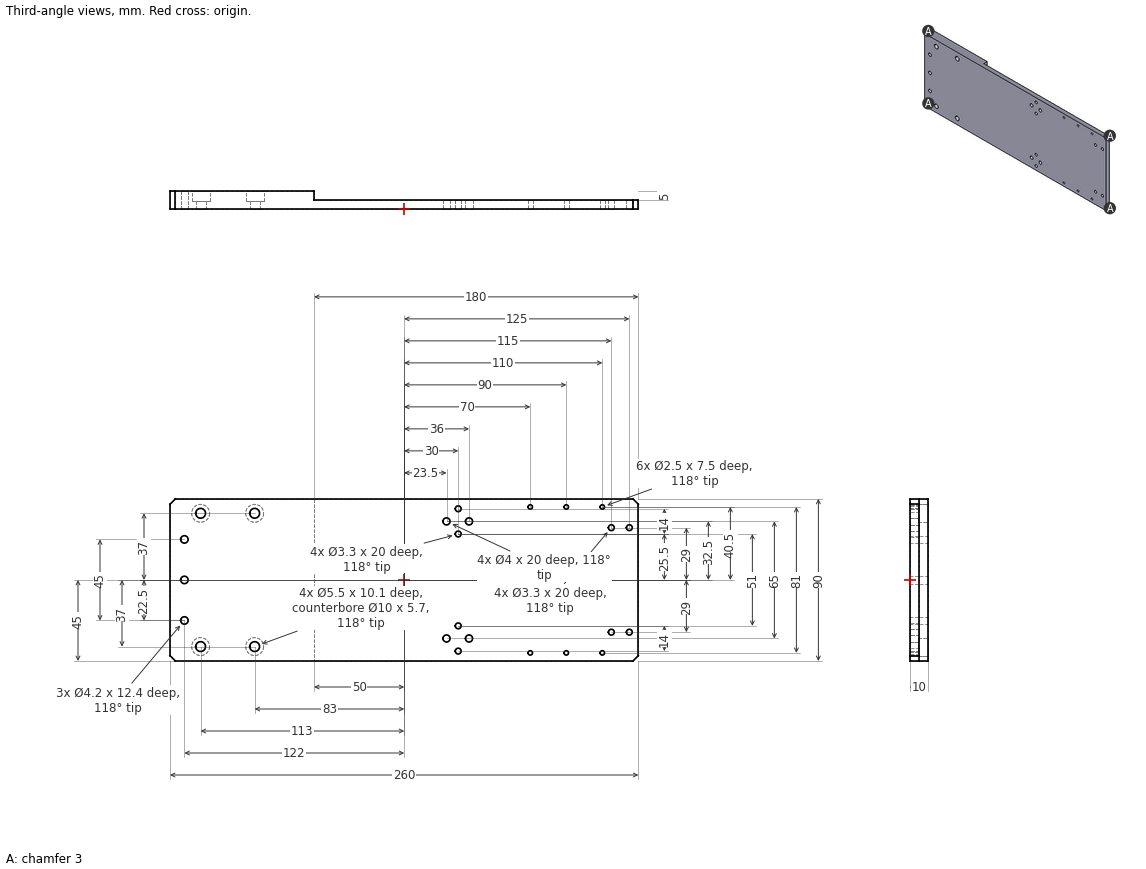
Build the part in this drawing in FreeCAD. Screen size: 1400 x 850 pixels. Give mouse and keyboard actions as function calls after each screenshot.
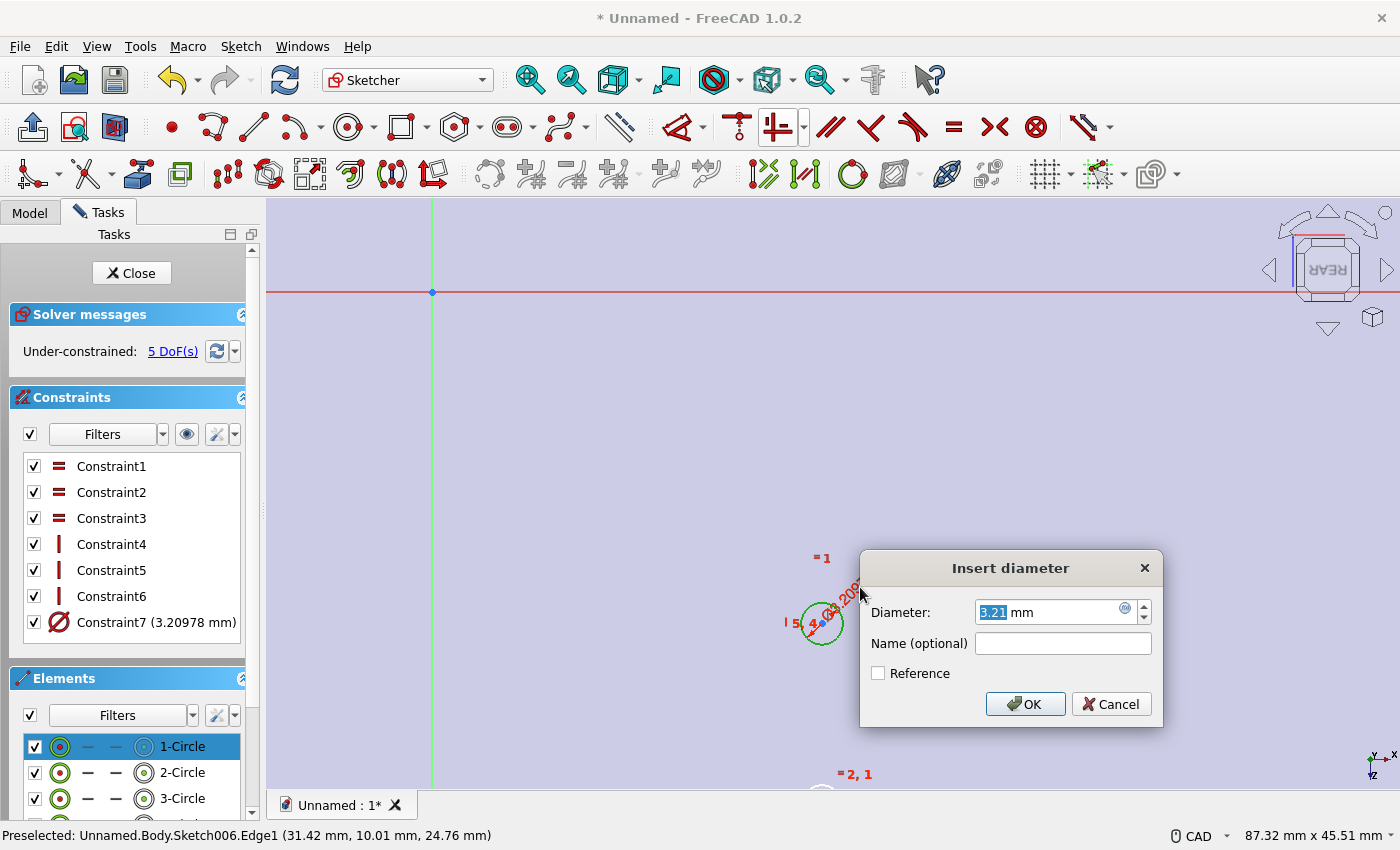
text(3.3)
key(Return)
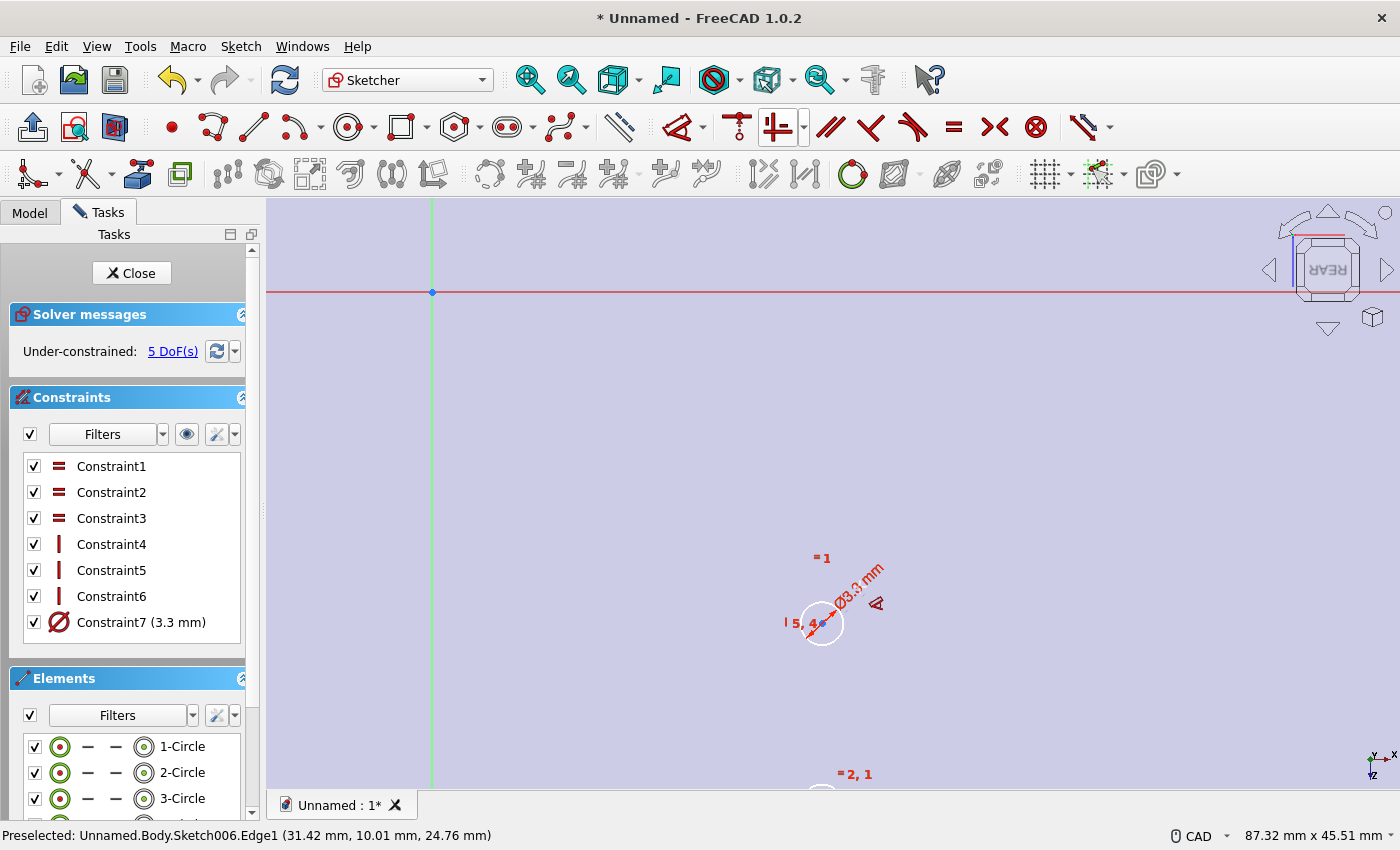
click(822, 624)
click(627, 658)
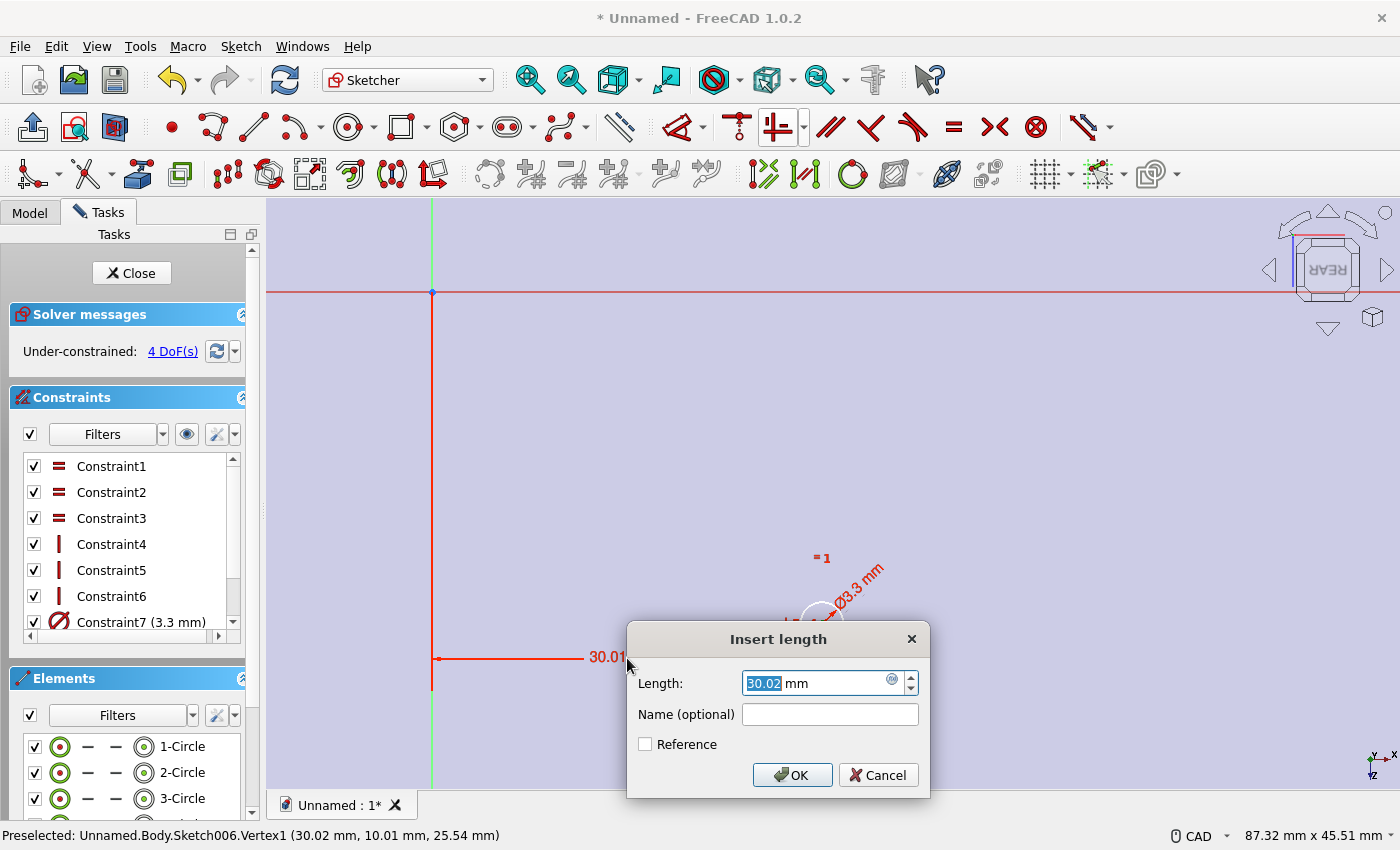
text(30)
key(Return)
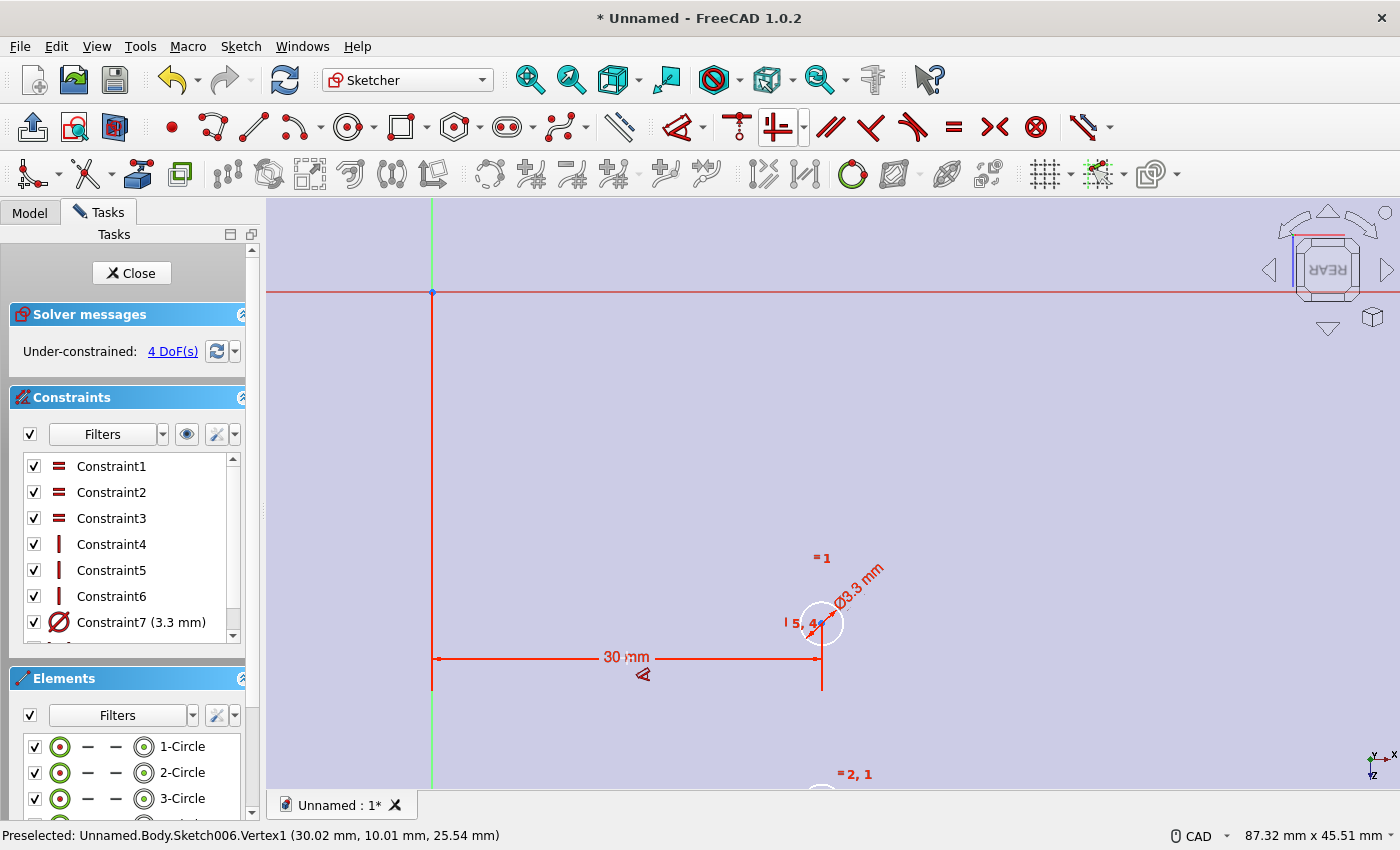
click(822, 624)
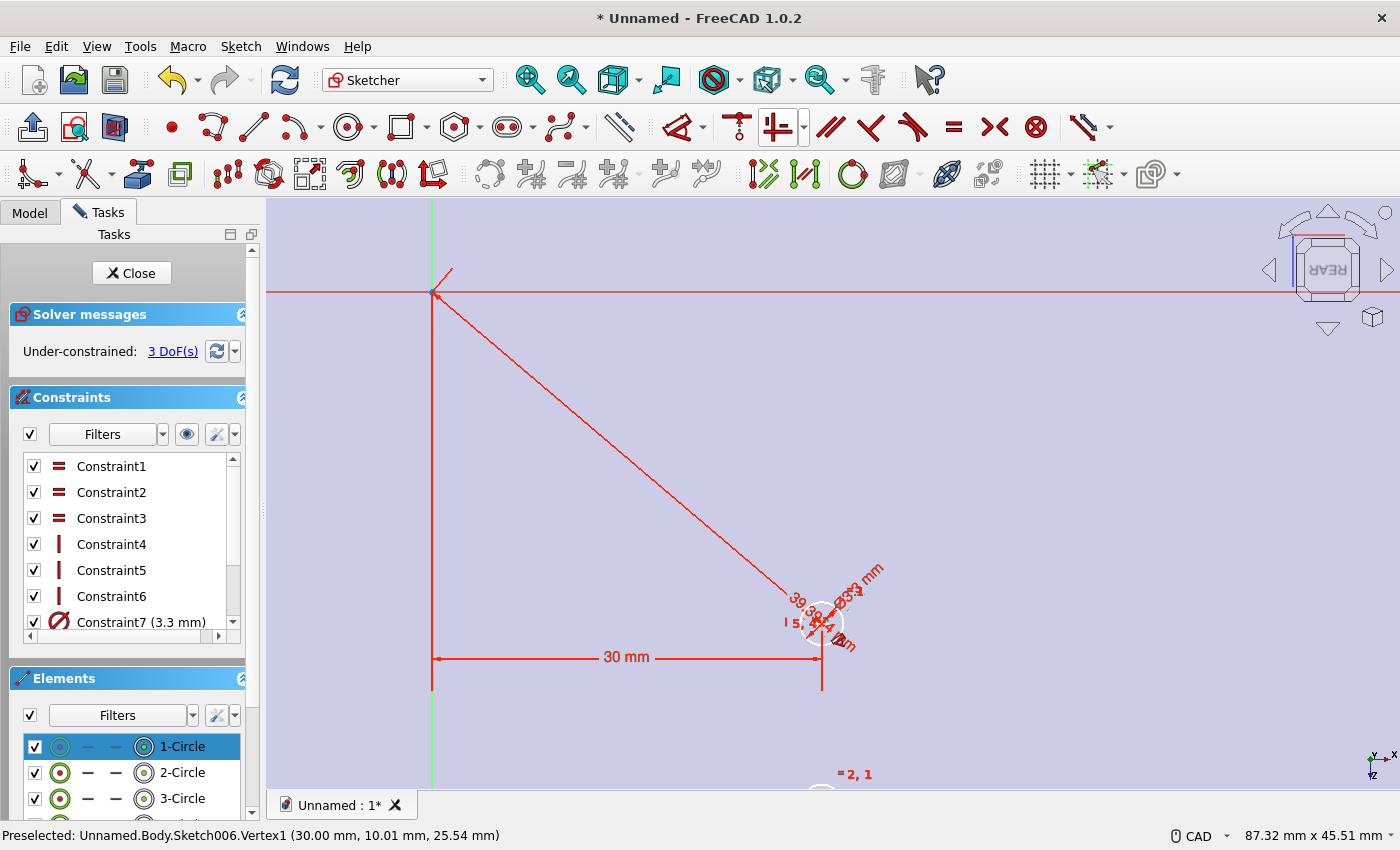
scroll(838, 611, down, 5)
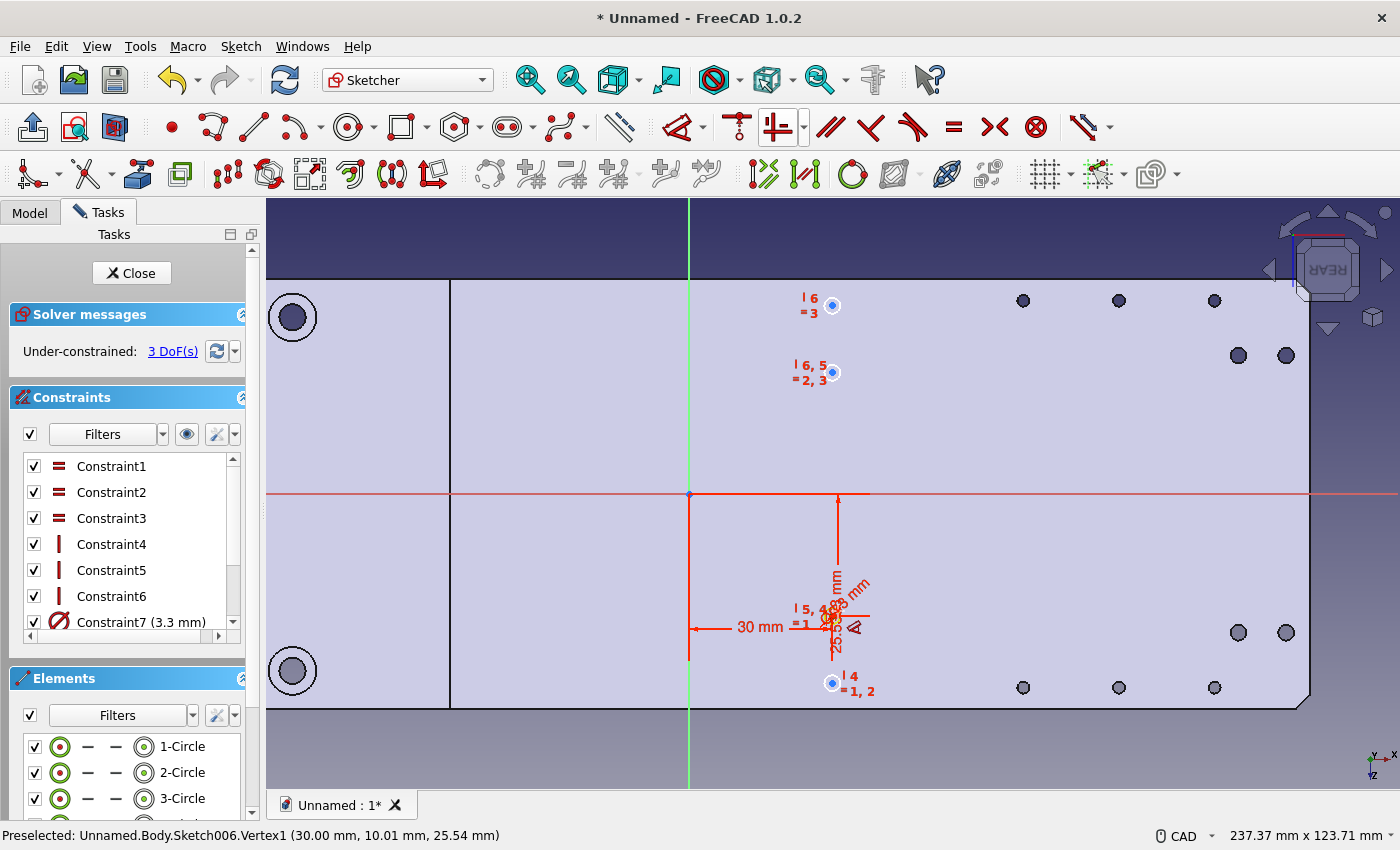
click(832, 683)
click(866, 650)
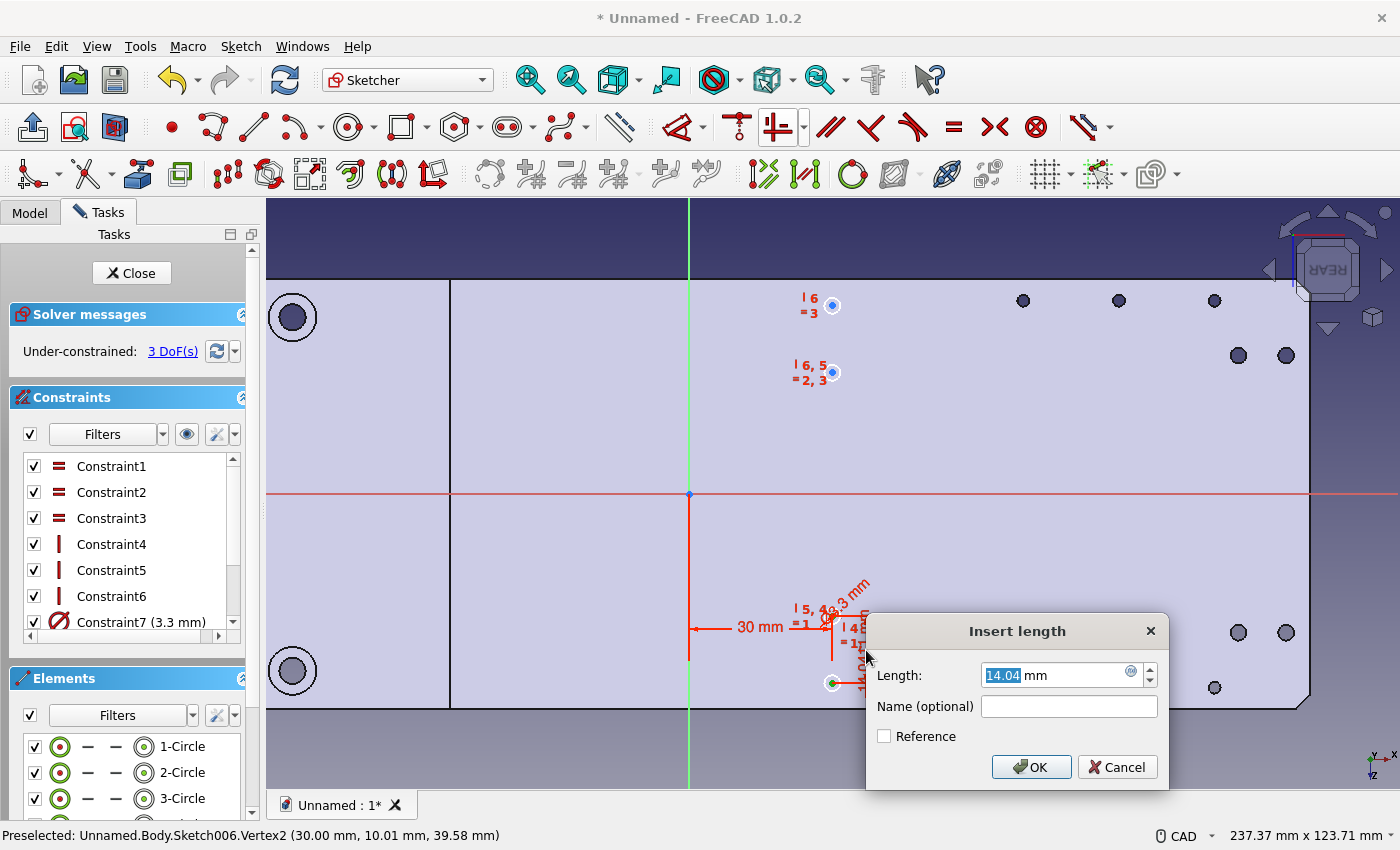
text(14)
key(Return)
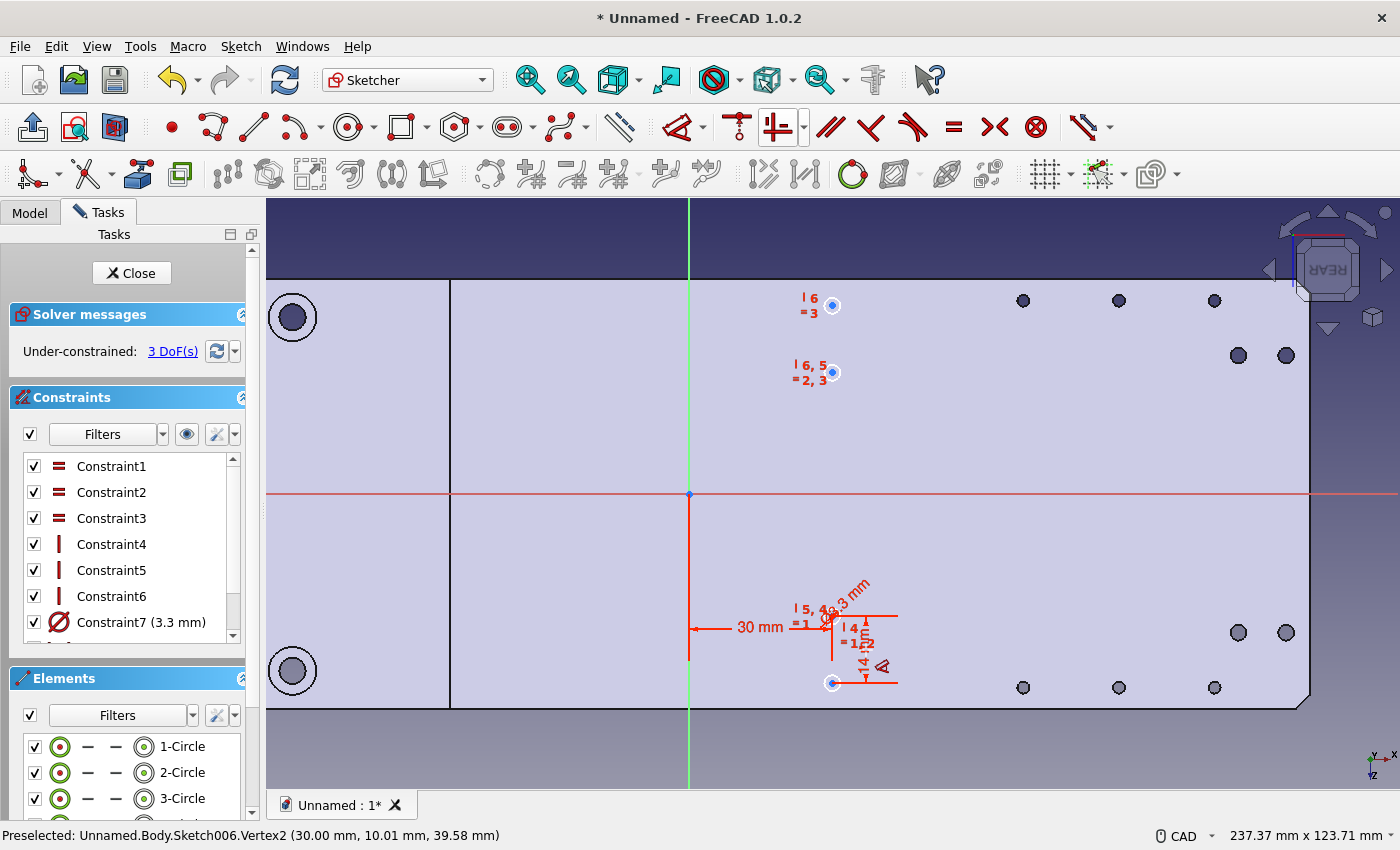
click(832, 616)